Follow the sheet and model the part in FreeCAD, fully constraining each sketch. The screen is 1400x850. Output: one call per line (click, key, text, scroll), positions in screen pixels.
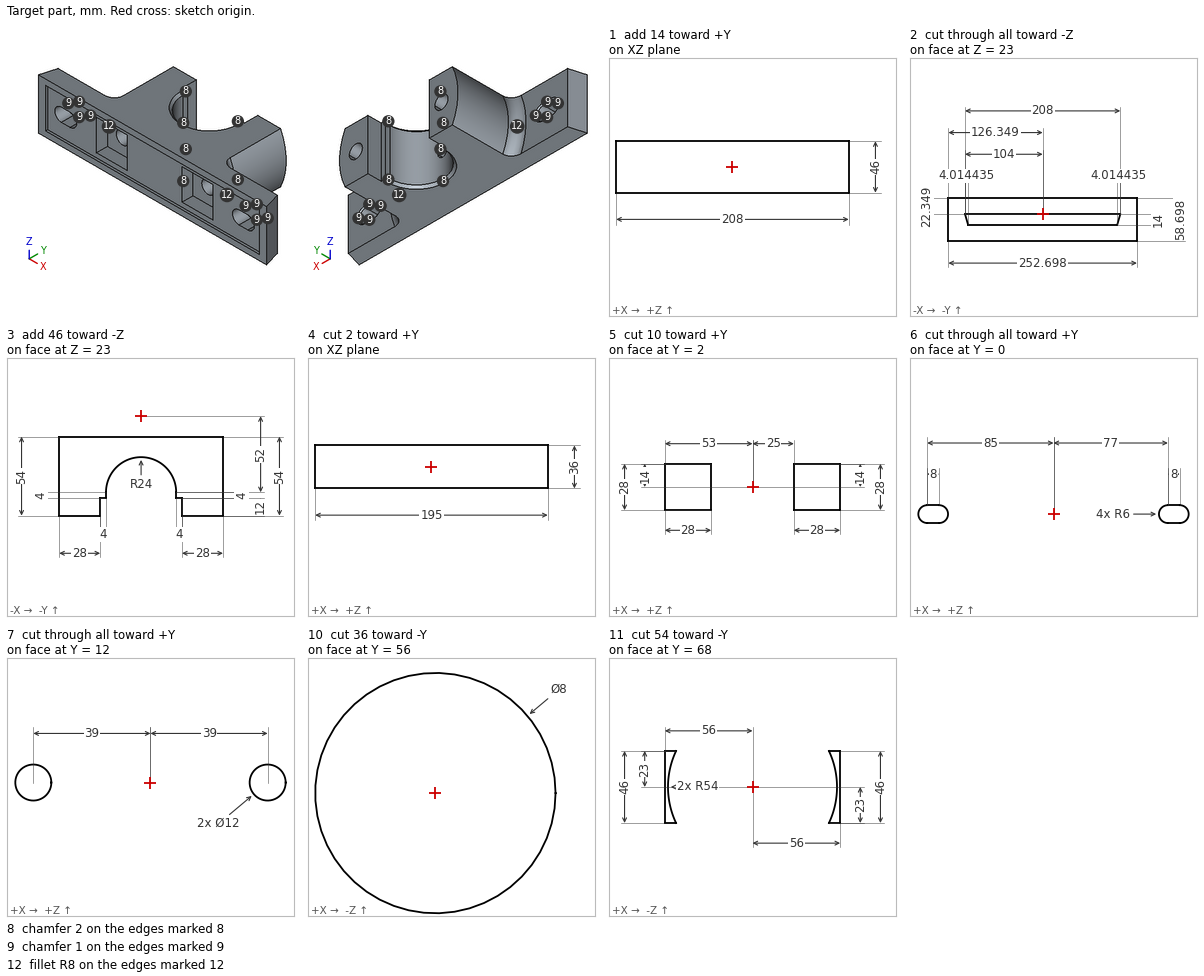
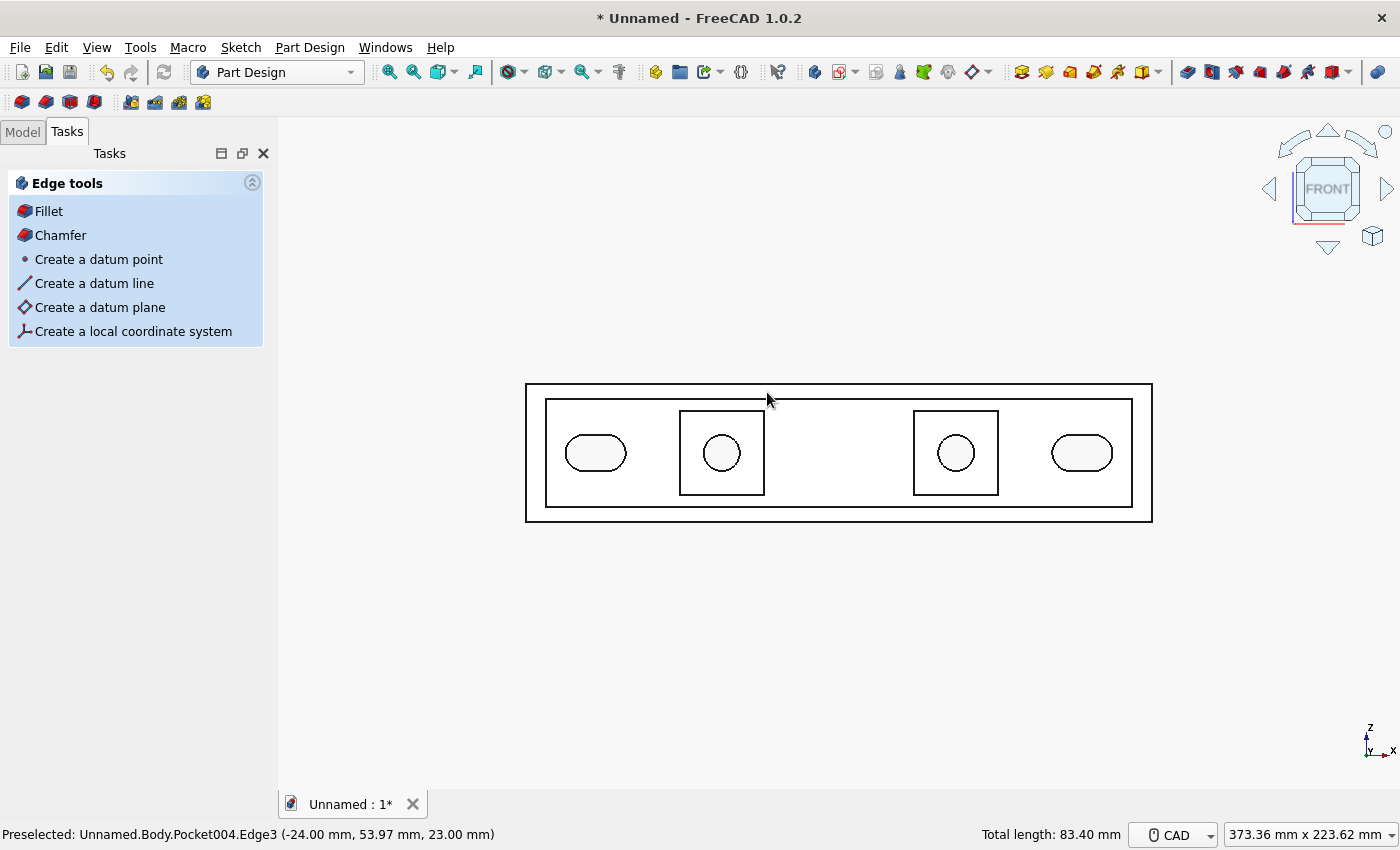
scroll(767, 521, up, 7)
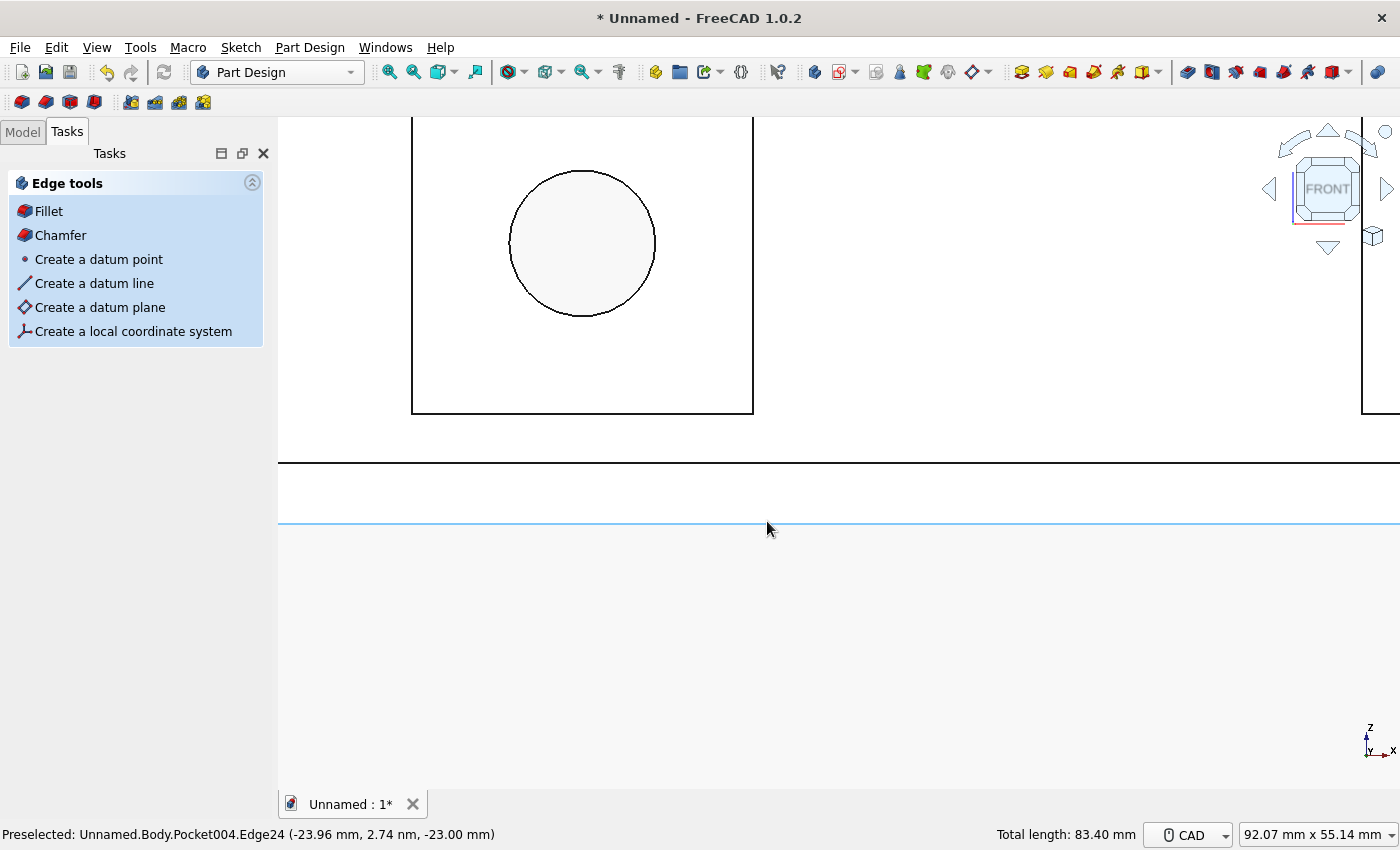
key(v)
key(f)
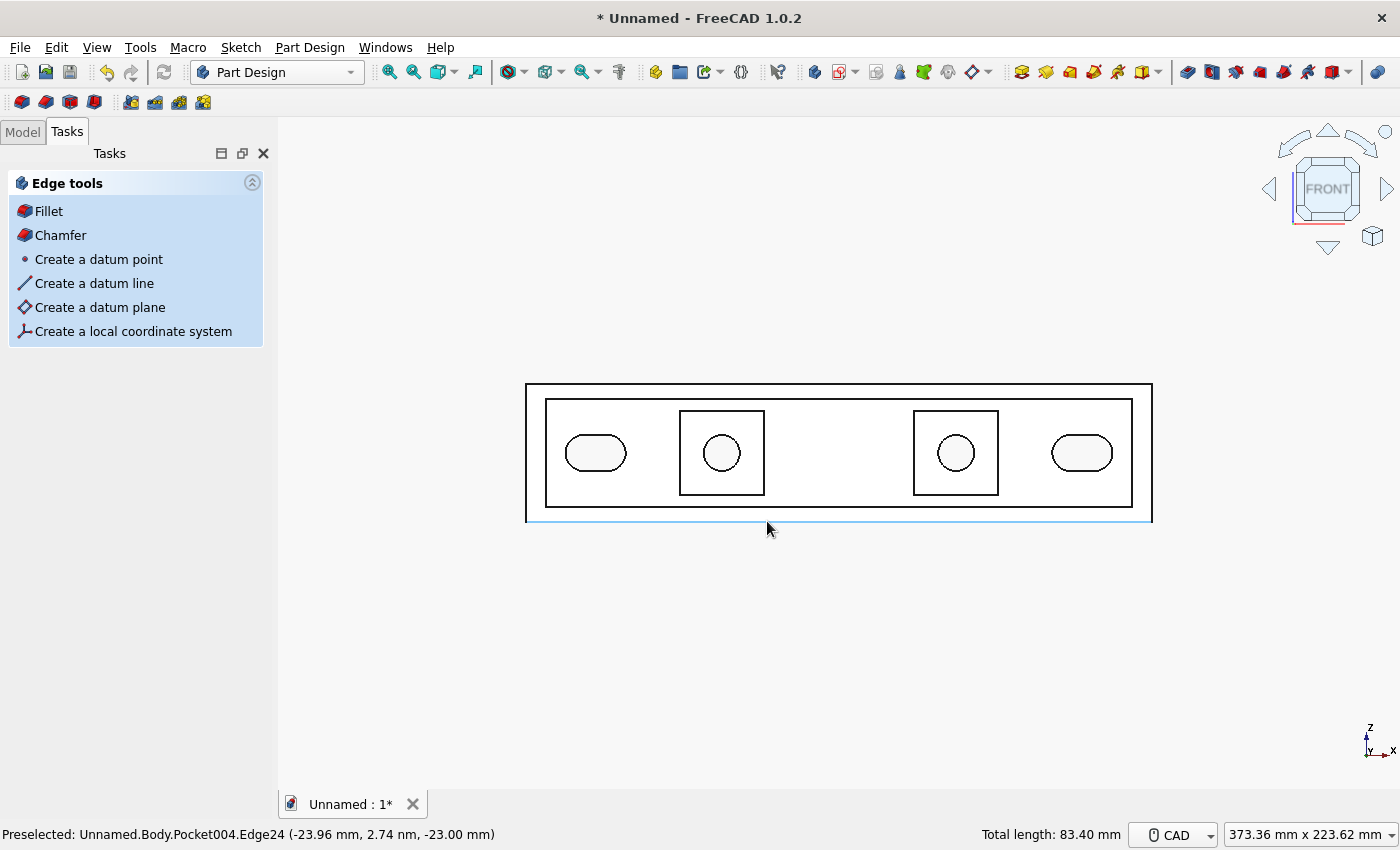
key(3)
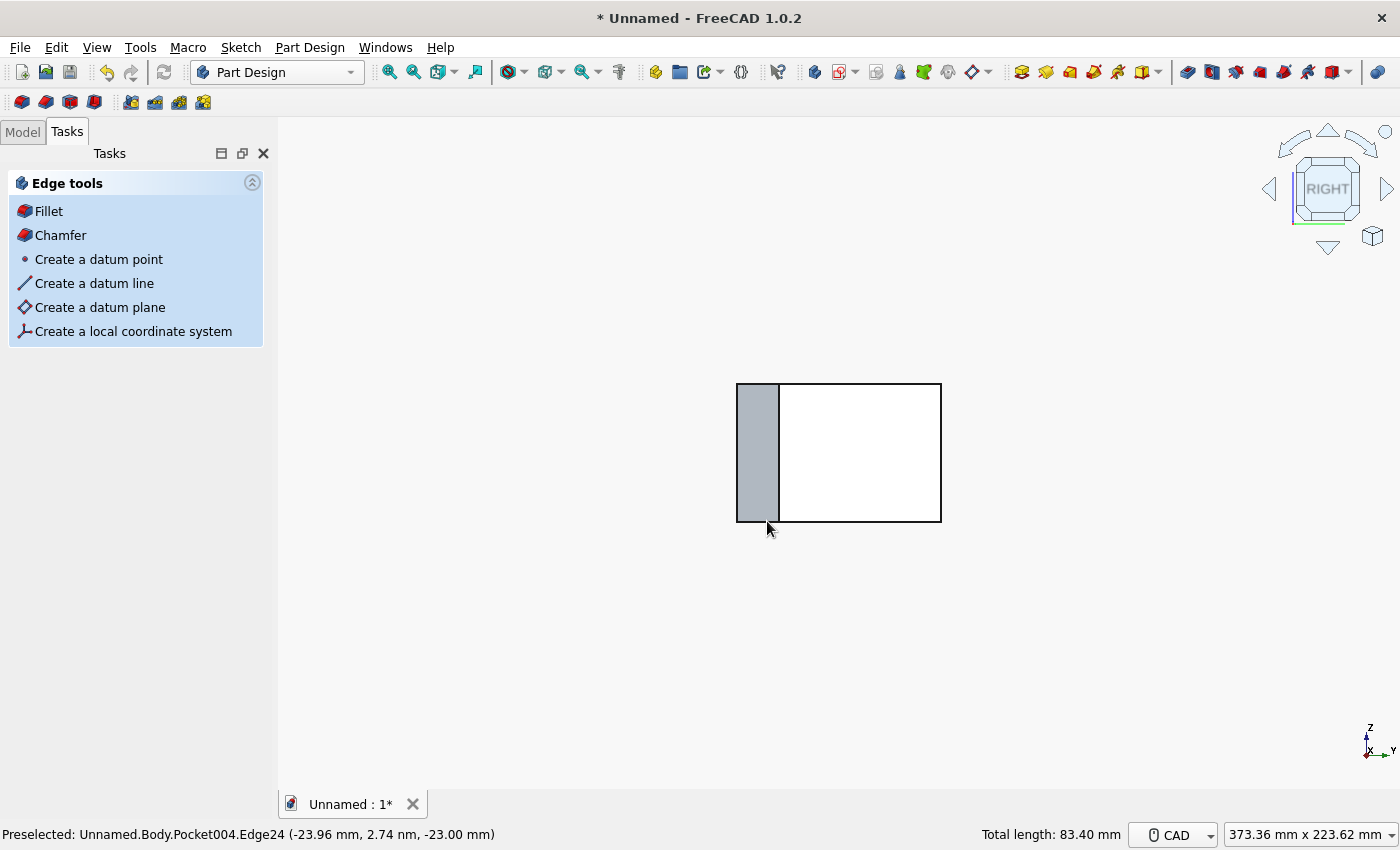
key(v)
key(f)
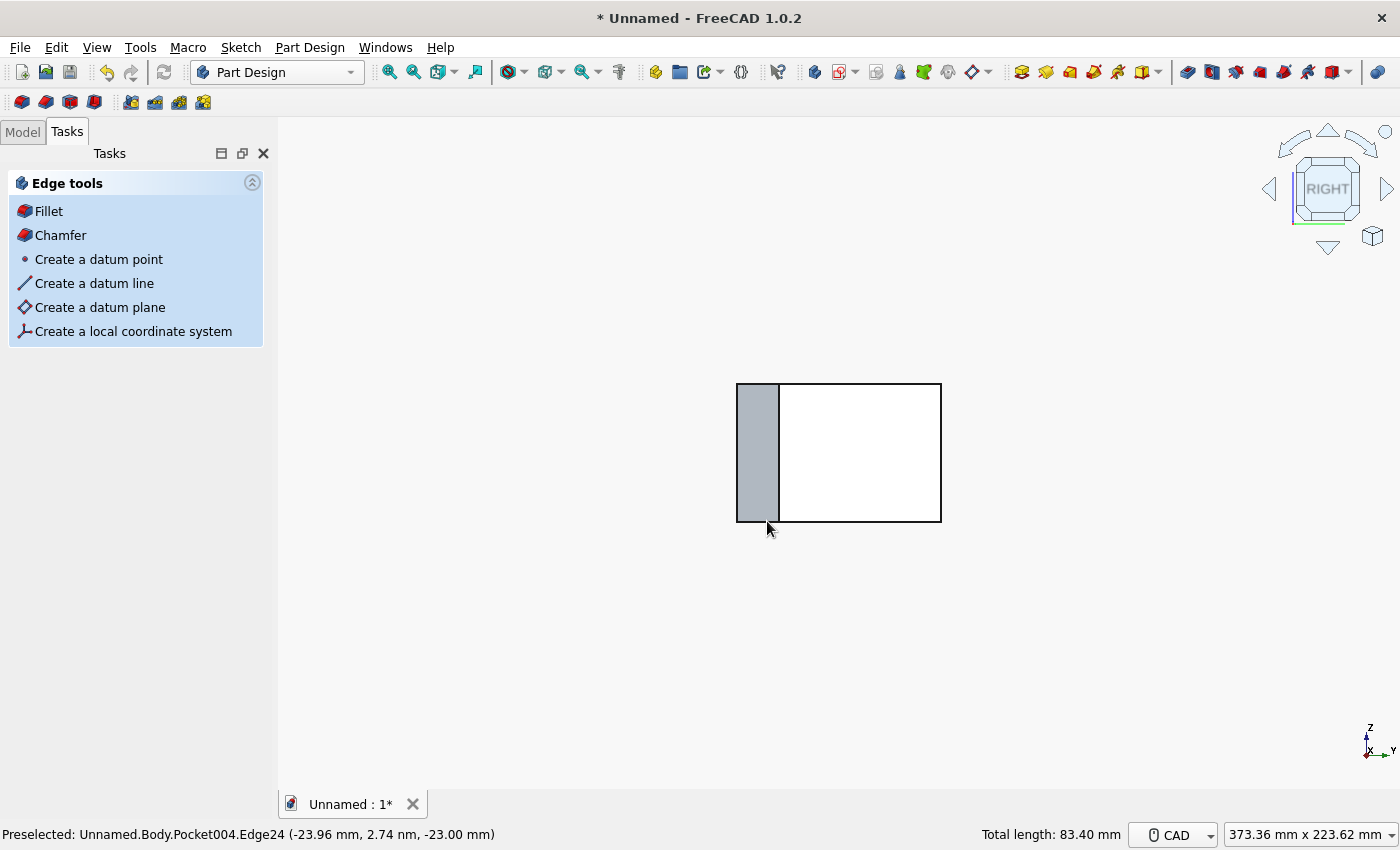
scroll(899, 521, up, 7)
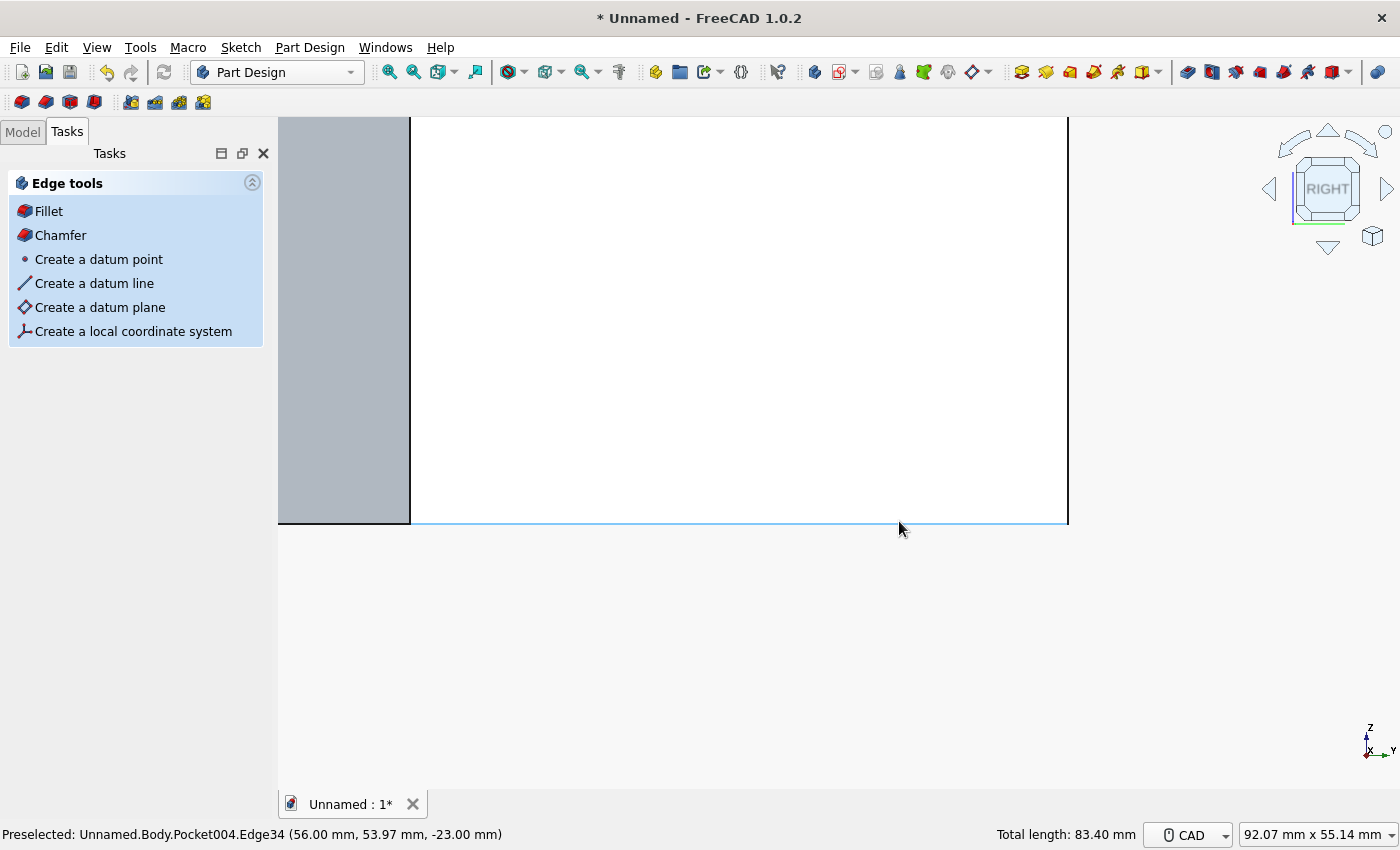
key(v)
key(f)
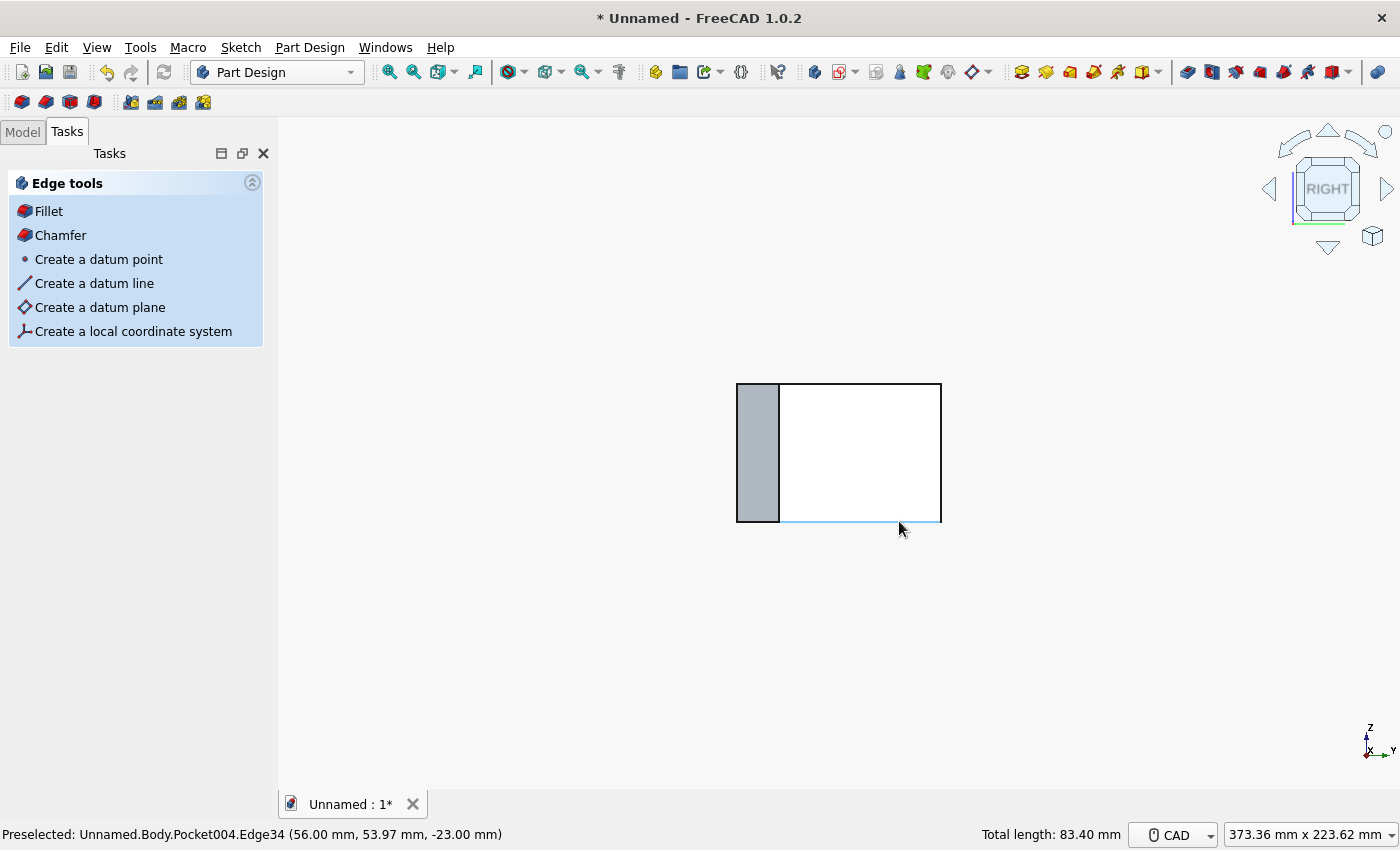
key(5)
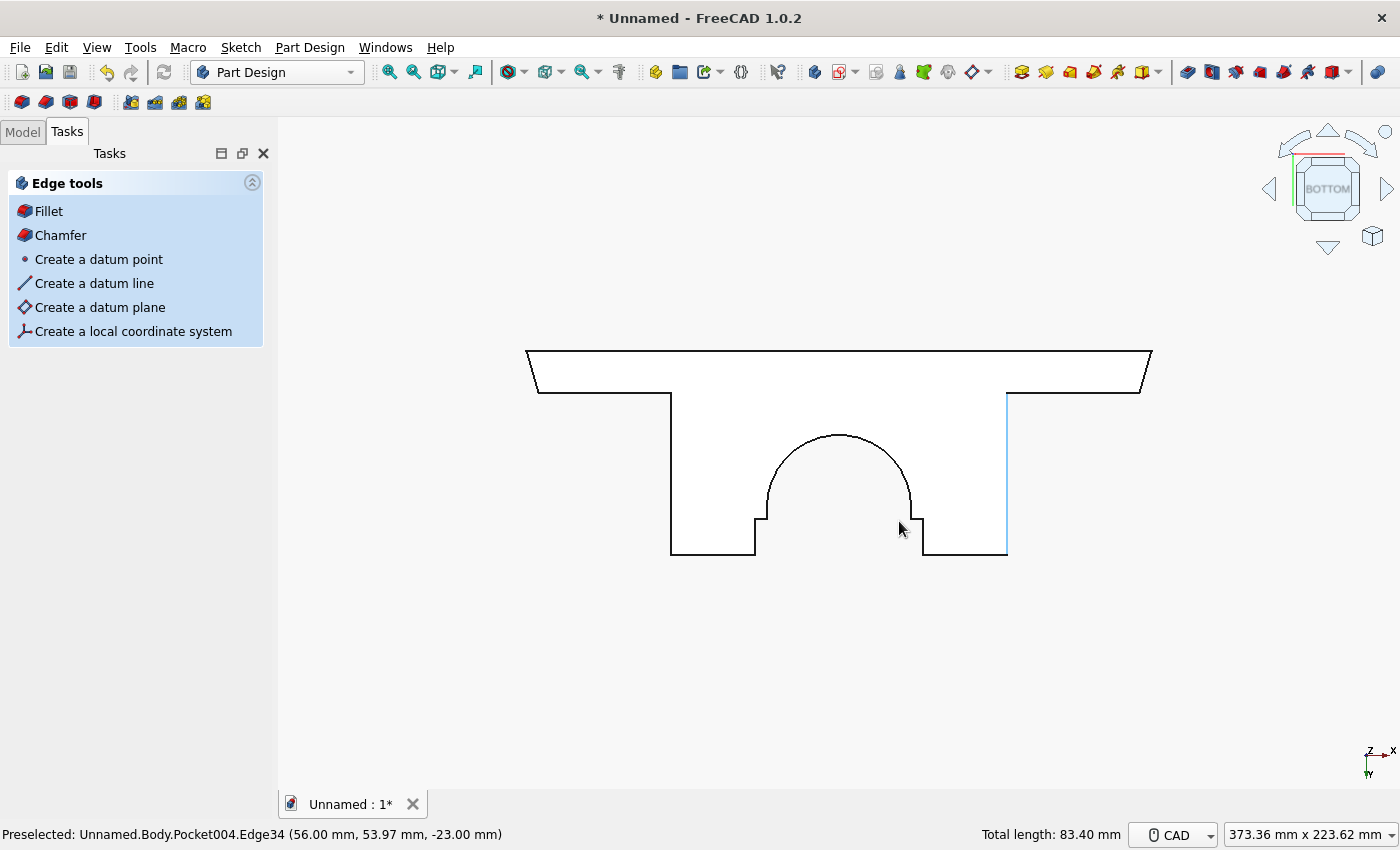
click(767, 513, ctrl)